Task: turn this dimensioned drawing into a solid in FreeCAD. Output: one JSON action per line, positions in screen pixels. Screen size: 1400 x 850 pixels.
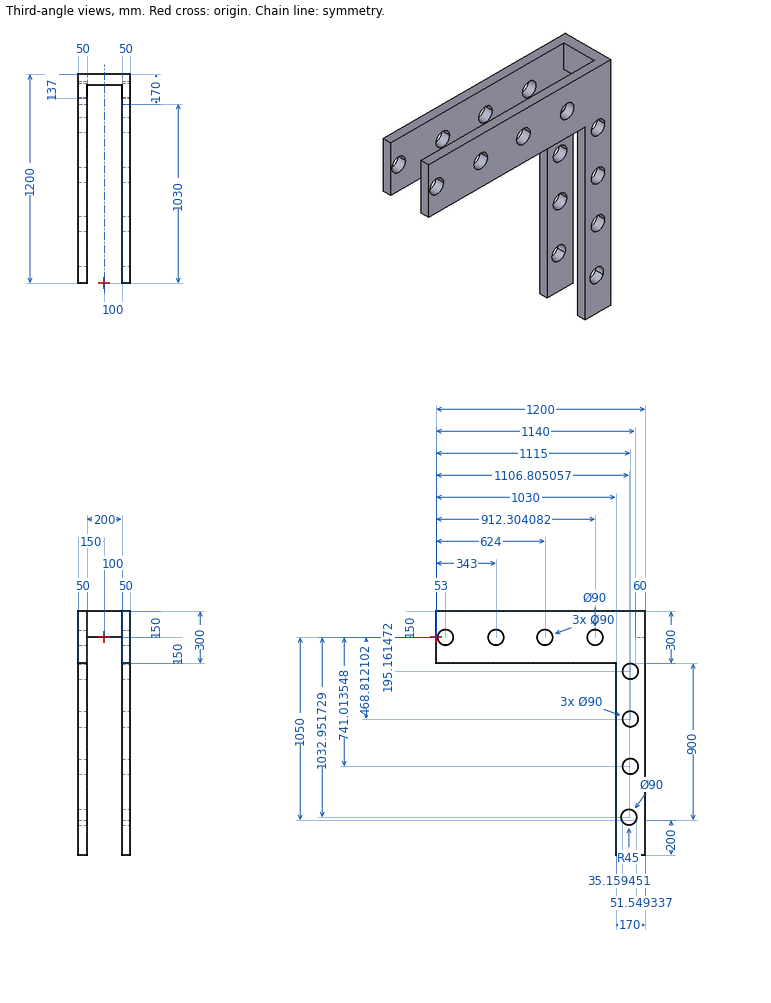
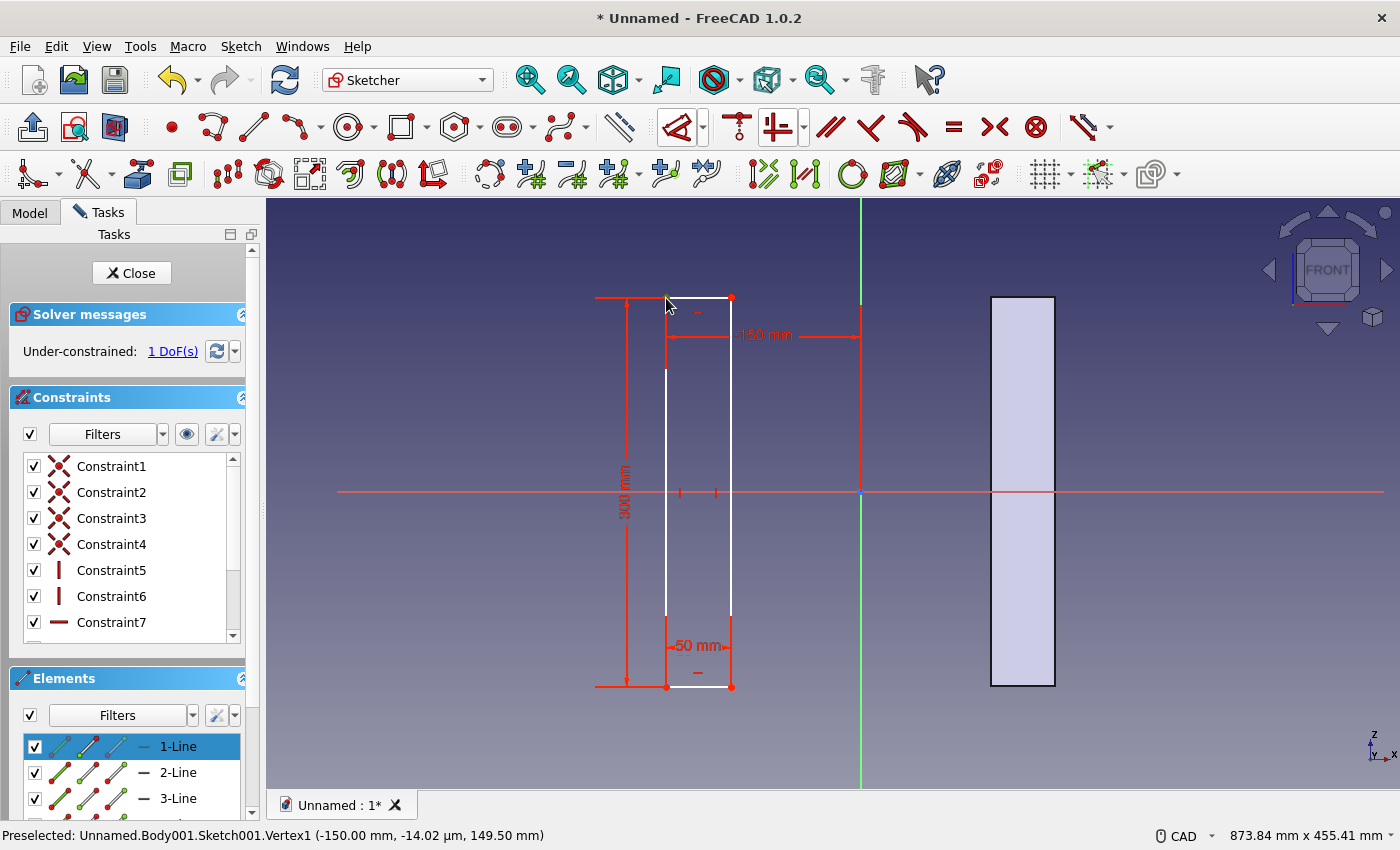
{"action": "left_click", "coordinate": [702, 128]}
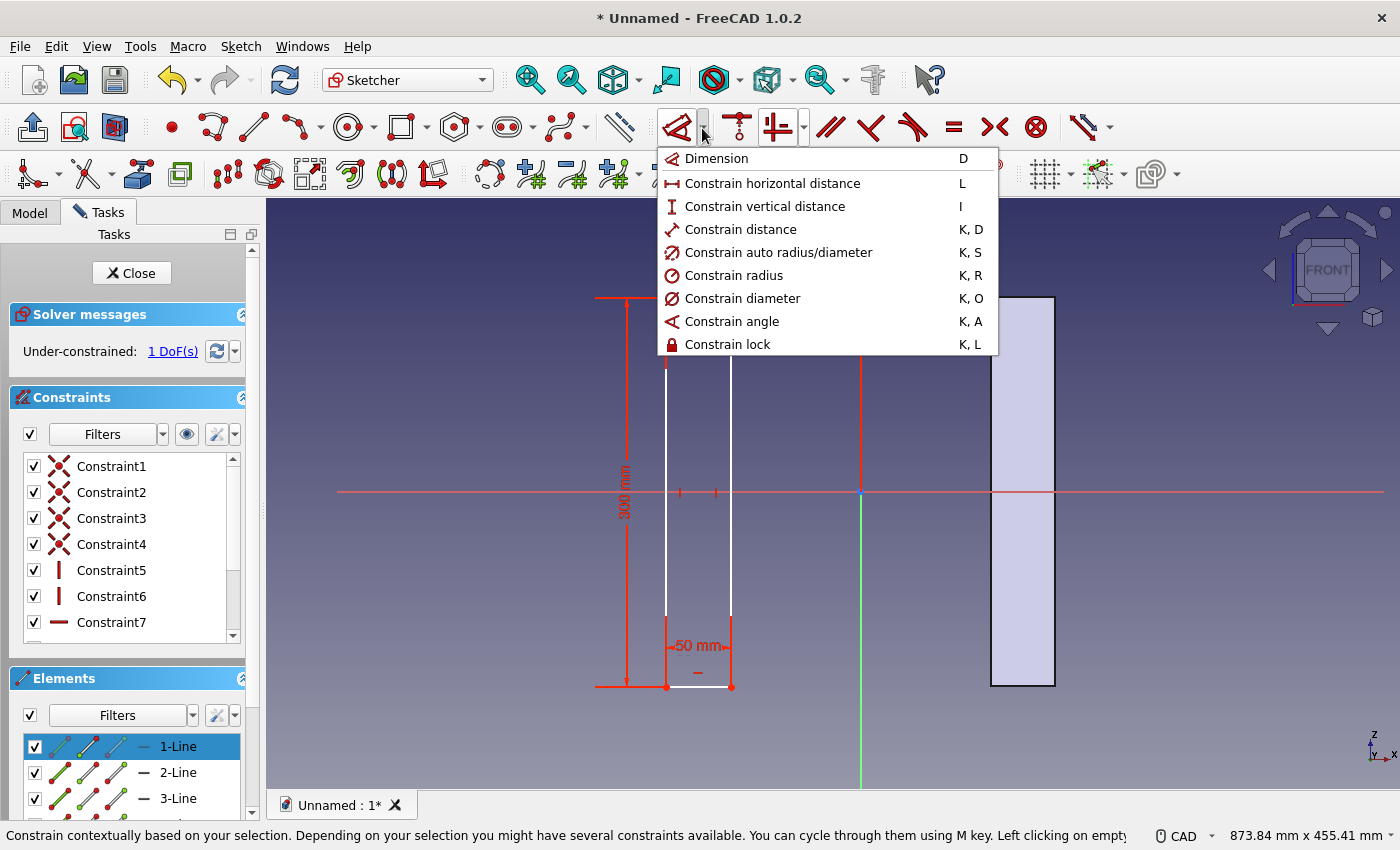
{"action": "left_click", "coordinate": [828, 206]}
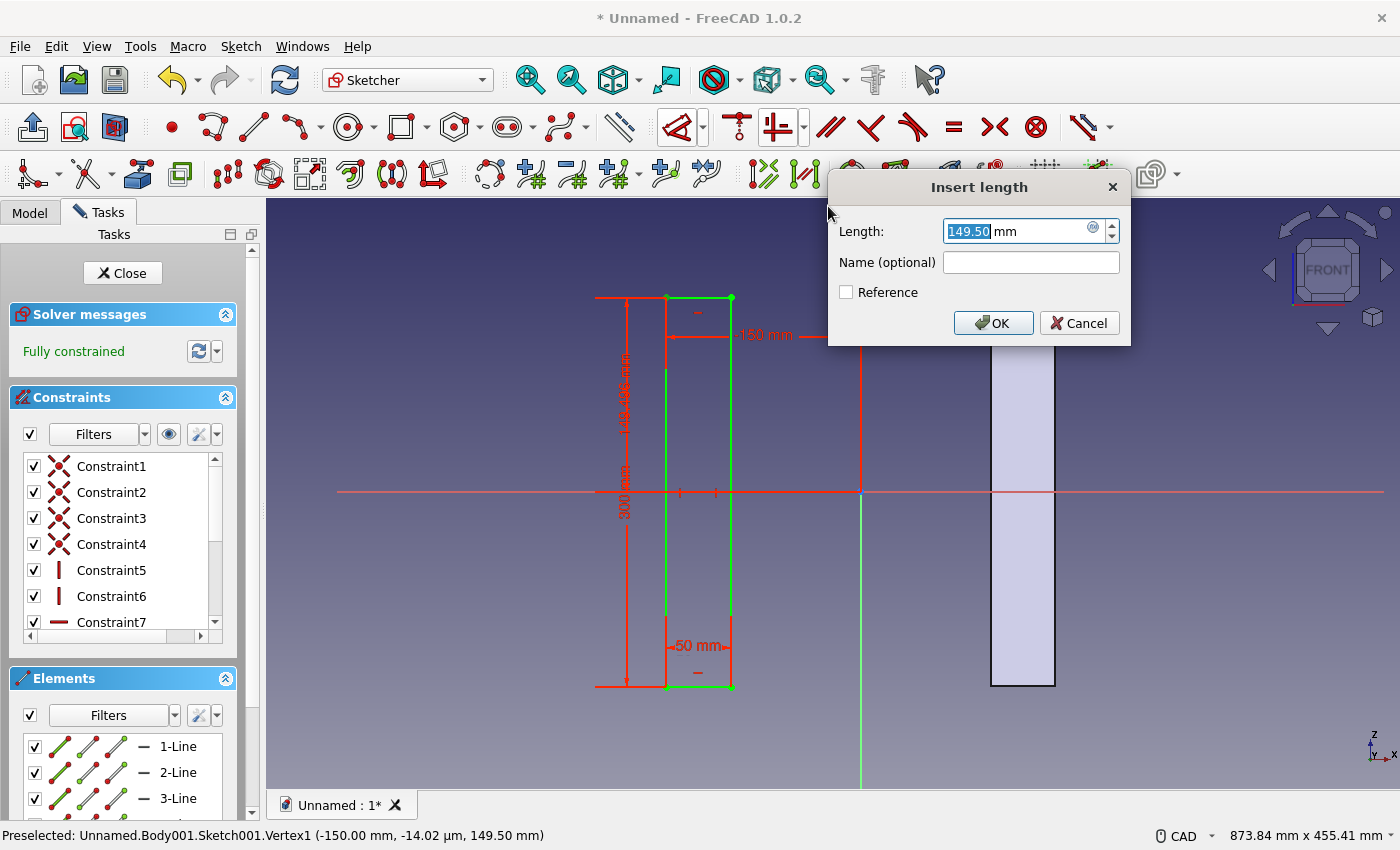
{"action": "type", "text": "150"}
{"action": "key", "text": "Return"}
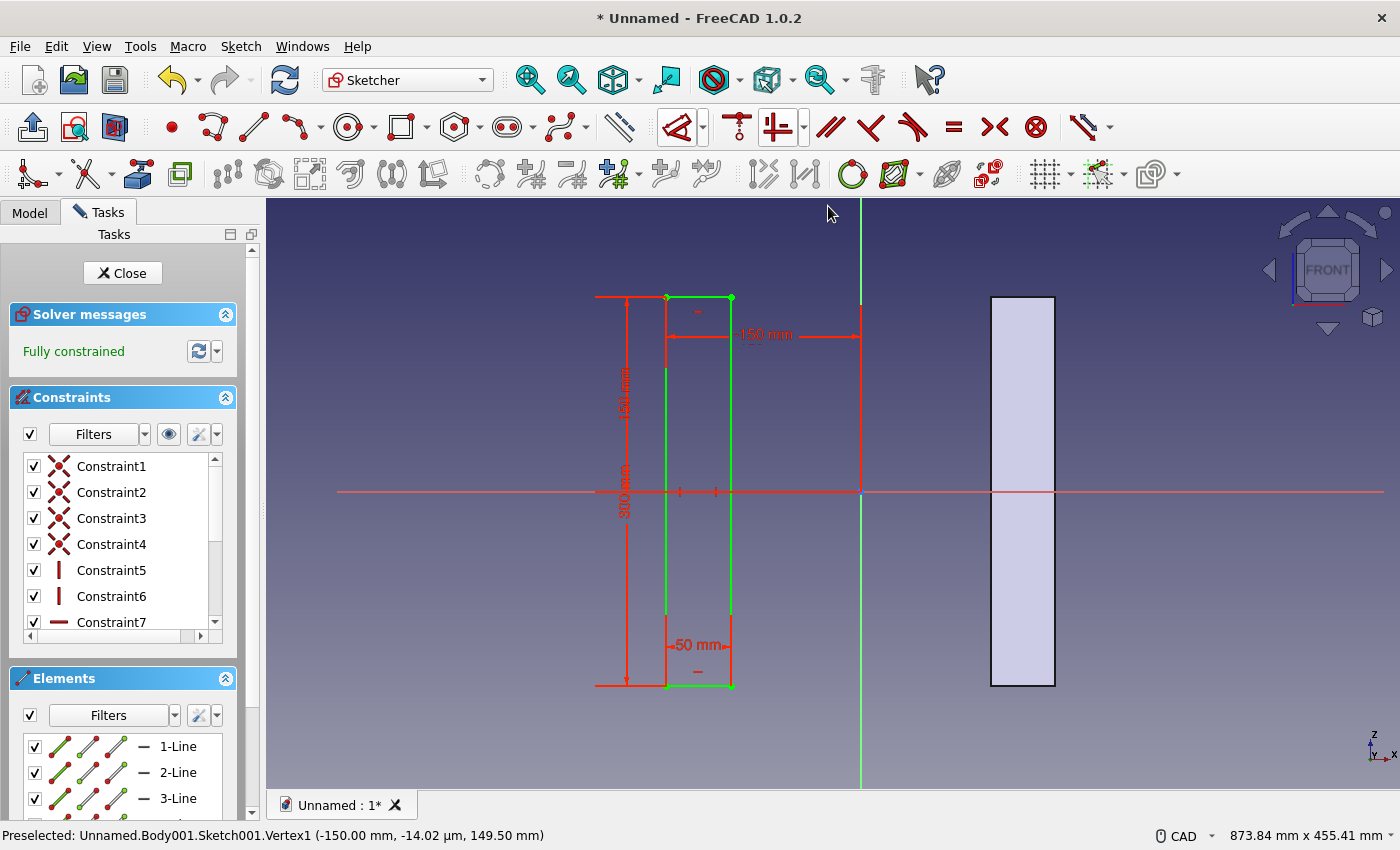
{"action": "left_click", "coordinate": [123, 273]}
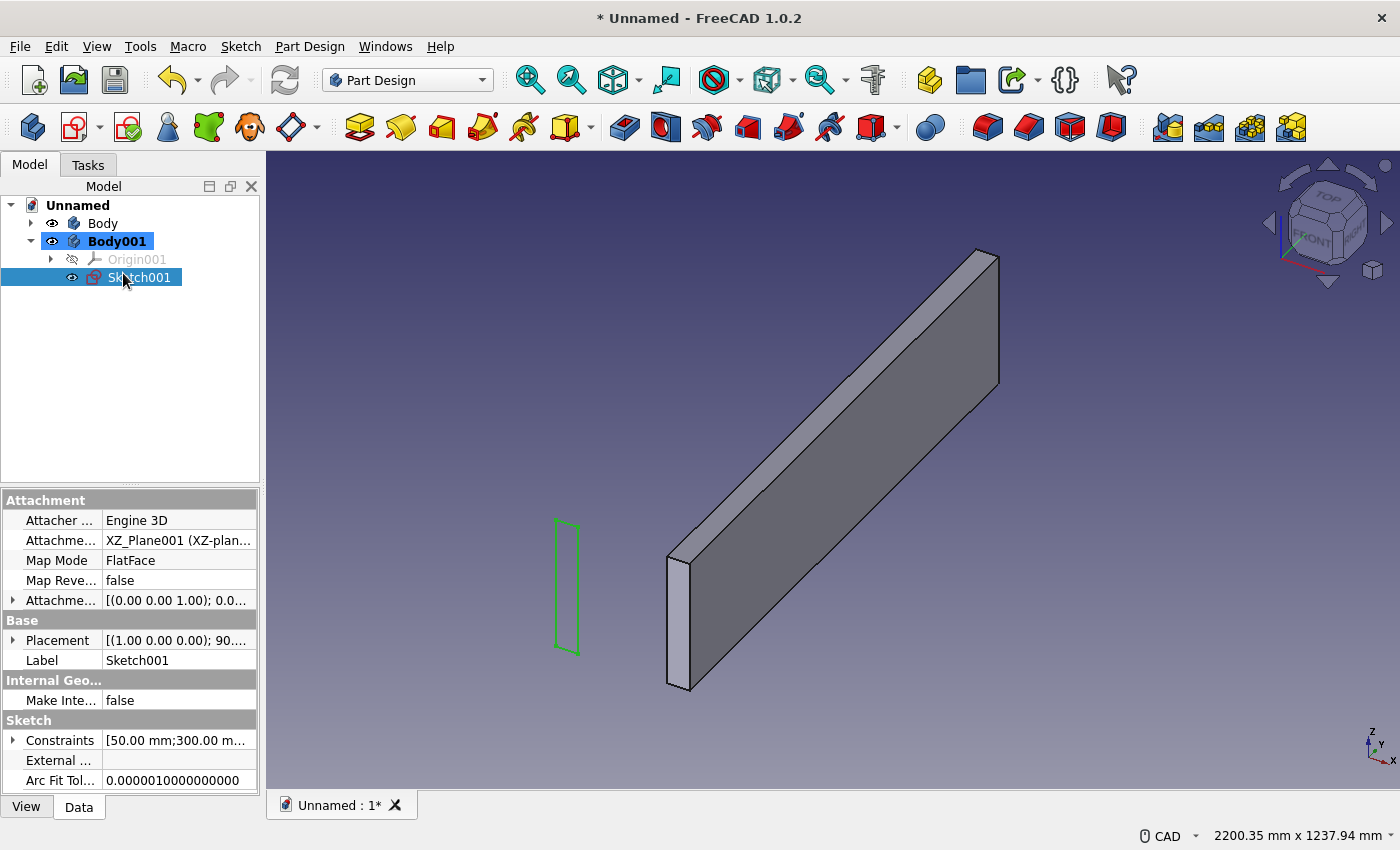
{"action": "left_click", "coordinate": [360, 128]}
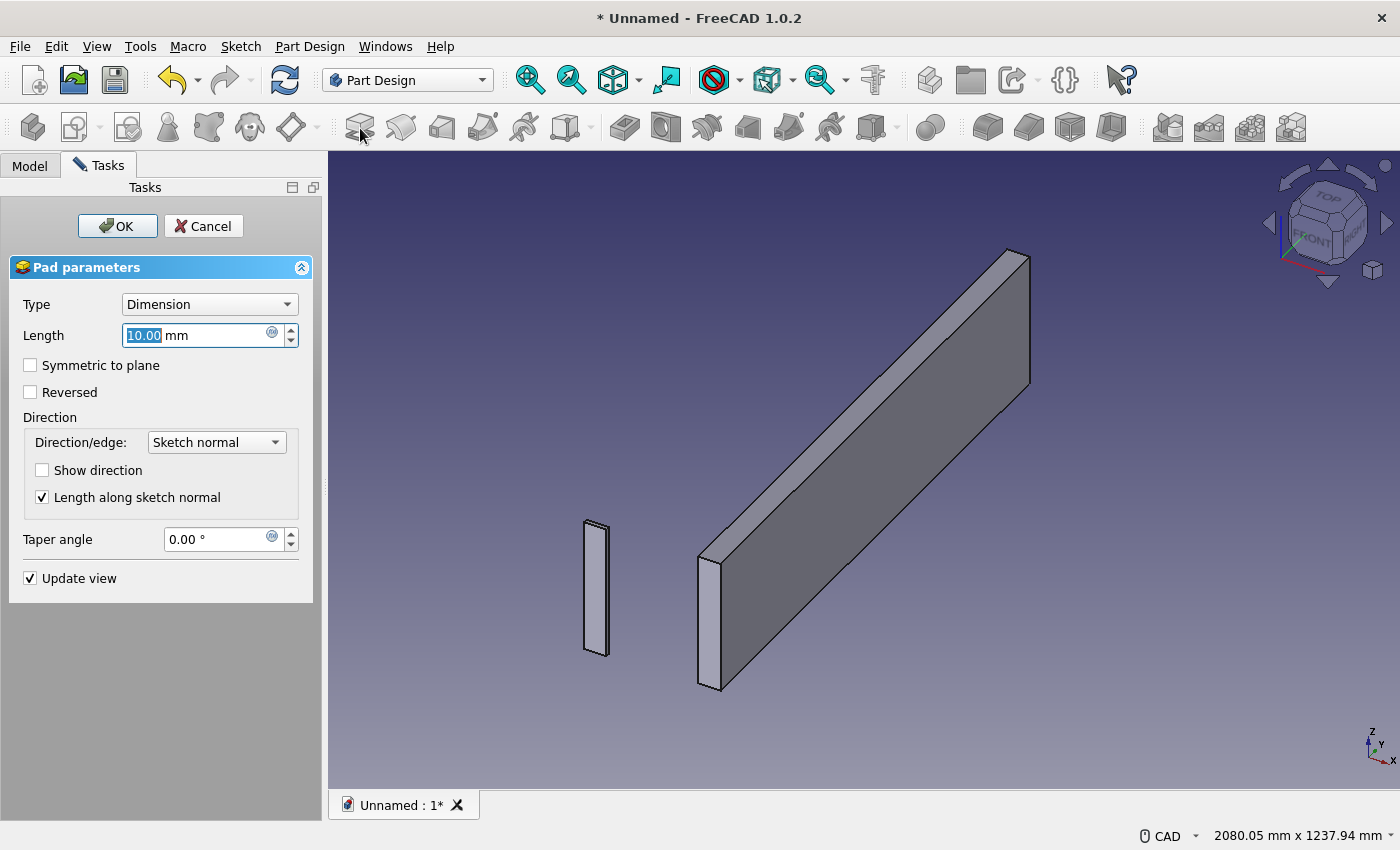
{"action": "type", "text": "1200"}
{"action": "key", "text": "Tab"}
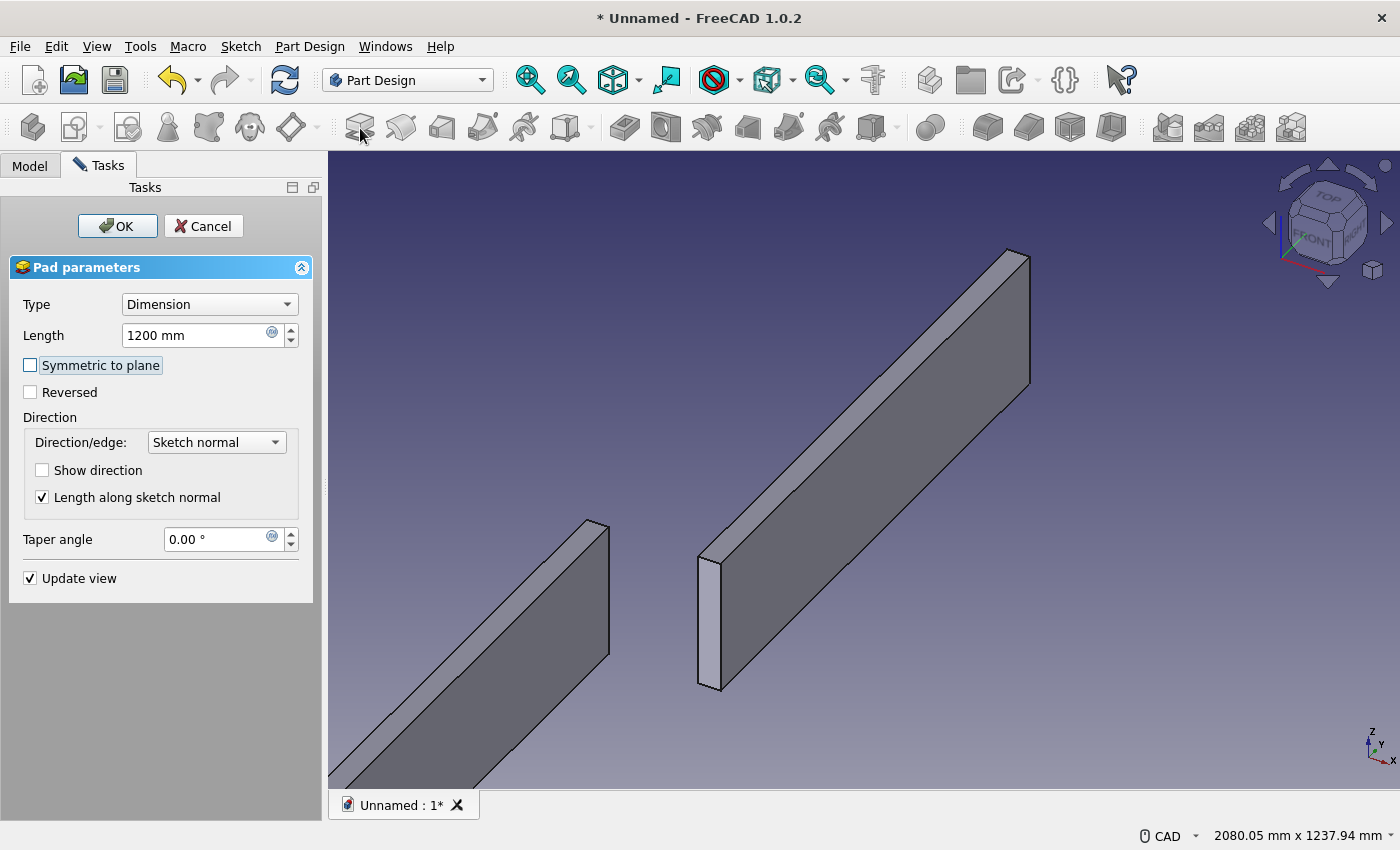
{"action": "left_click", "coordinate": [31, 392]}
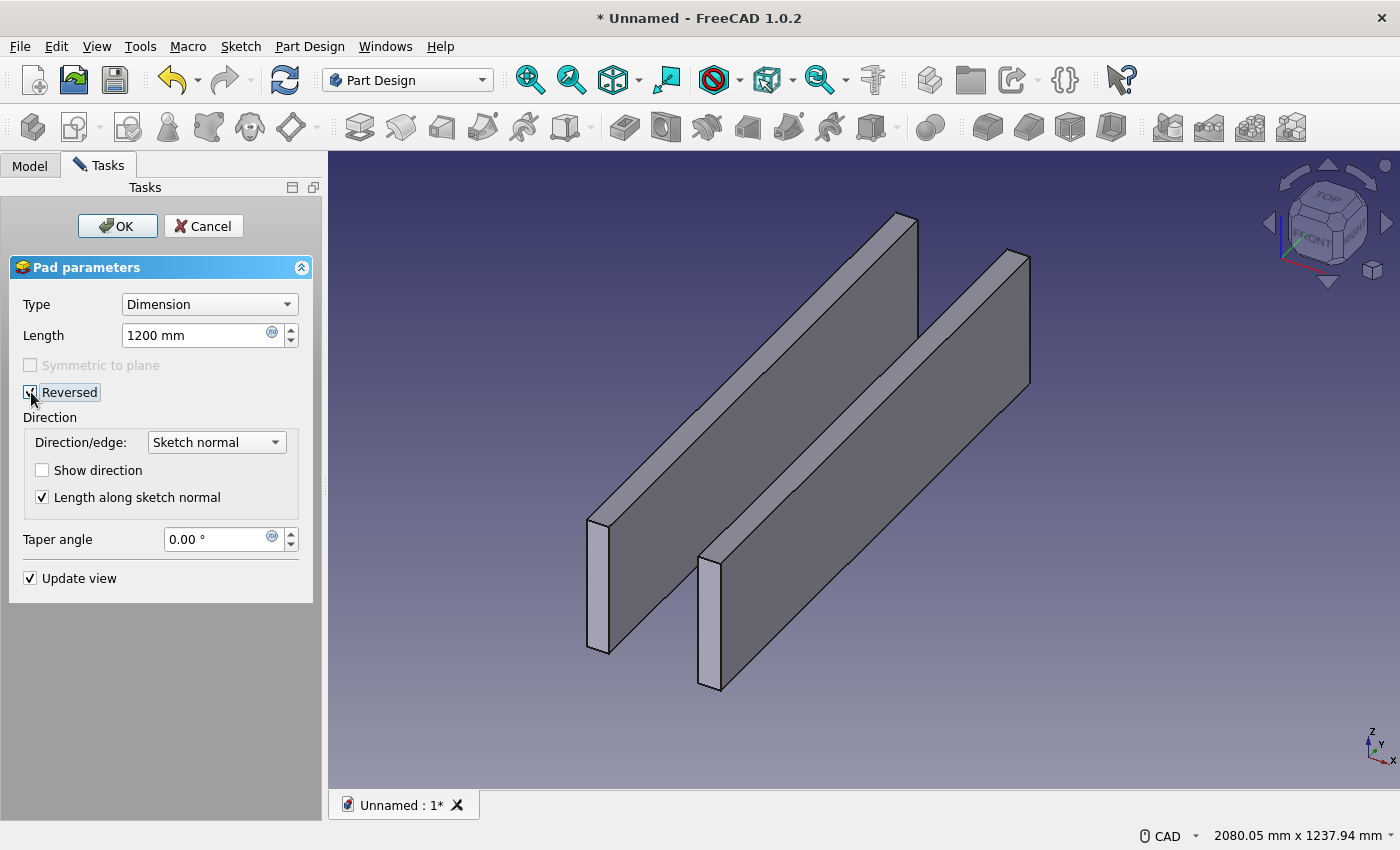
{"action": "left_click", "coordinate": [118, 226]}